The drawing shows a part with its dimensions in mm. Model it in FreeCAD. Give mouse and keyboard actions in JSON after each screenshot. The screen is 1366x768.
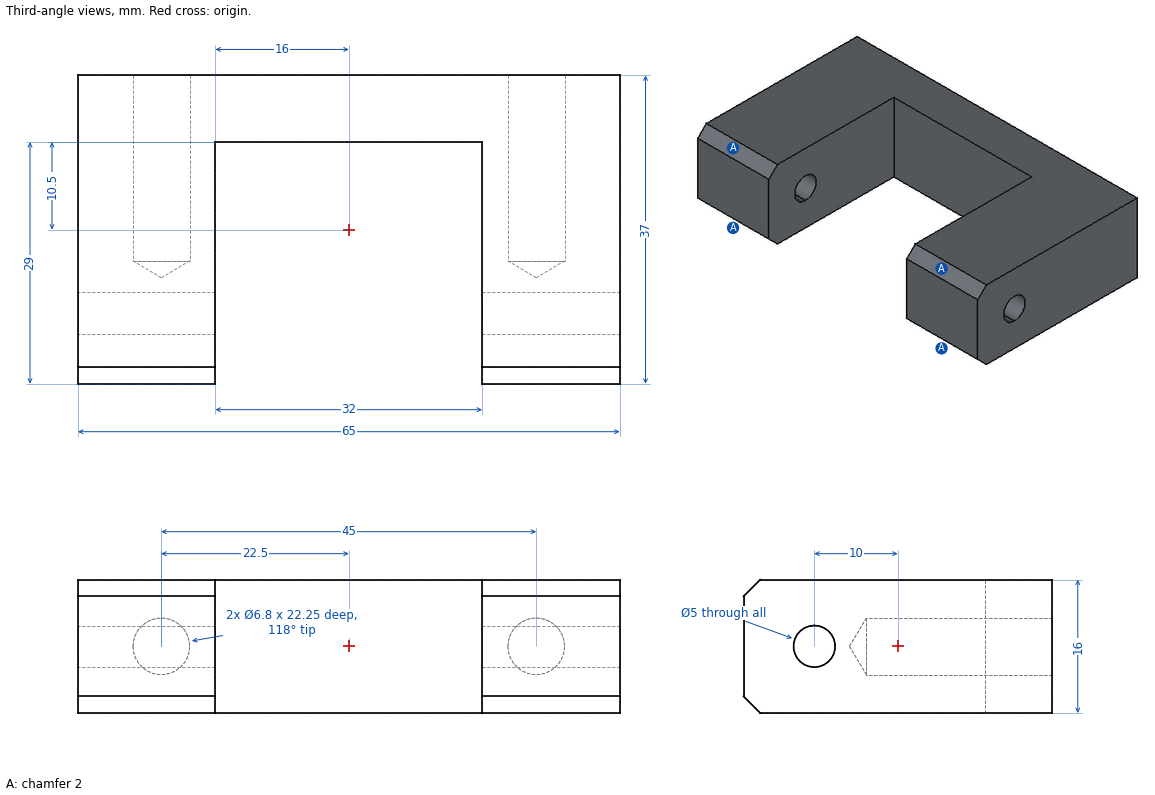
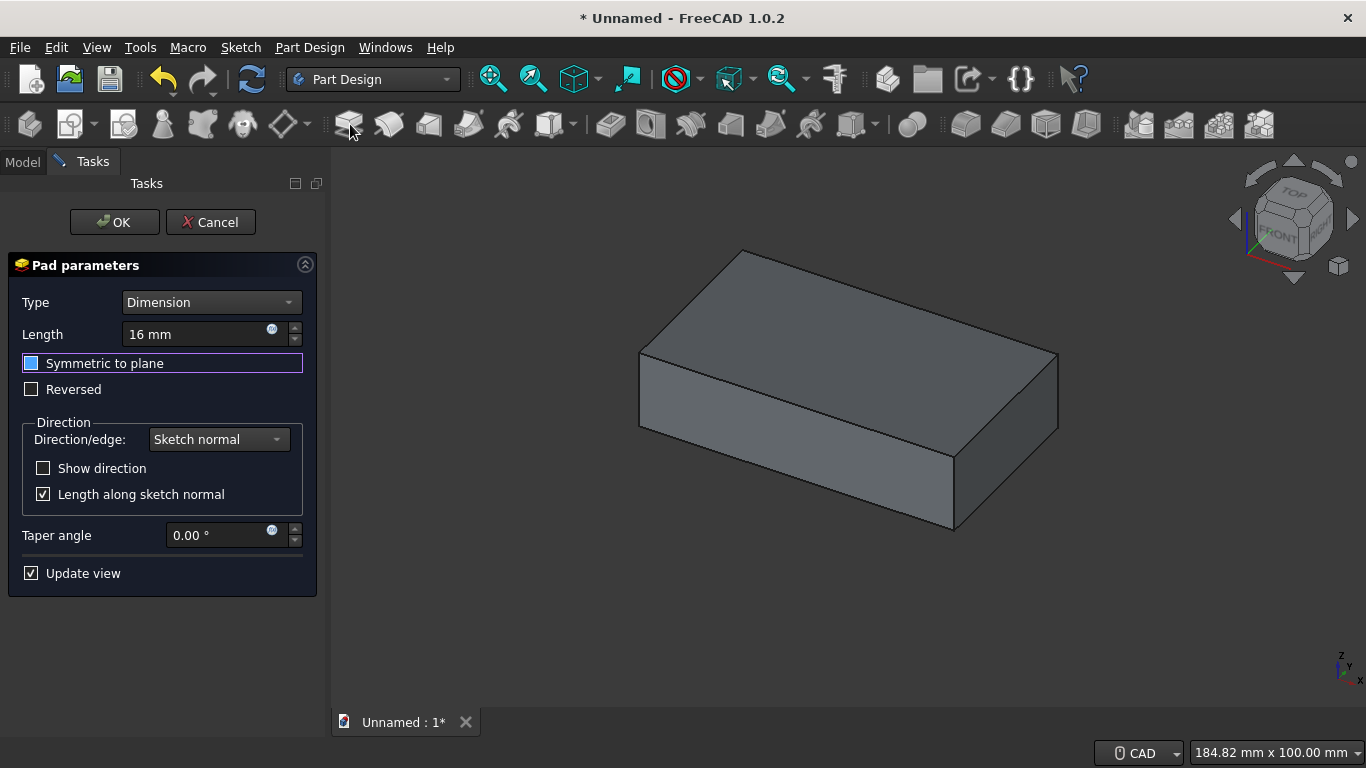
{"action": "left_click", "coordinate": [30, 363]}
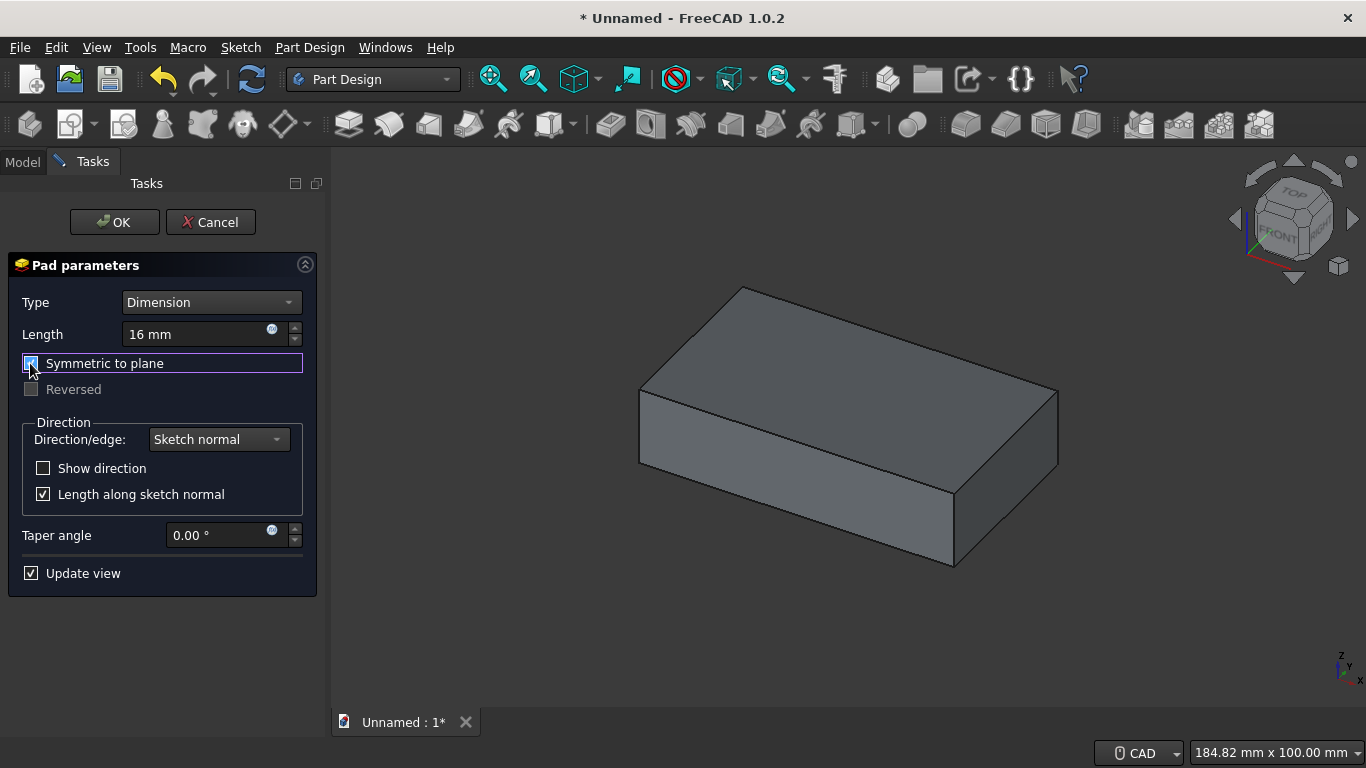
{"action": "left_click", "coordinate": [115, 222]}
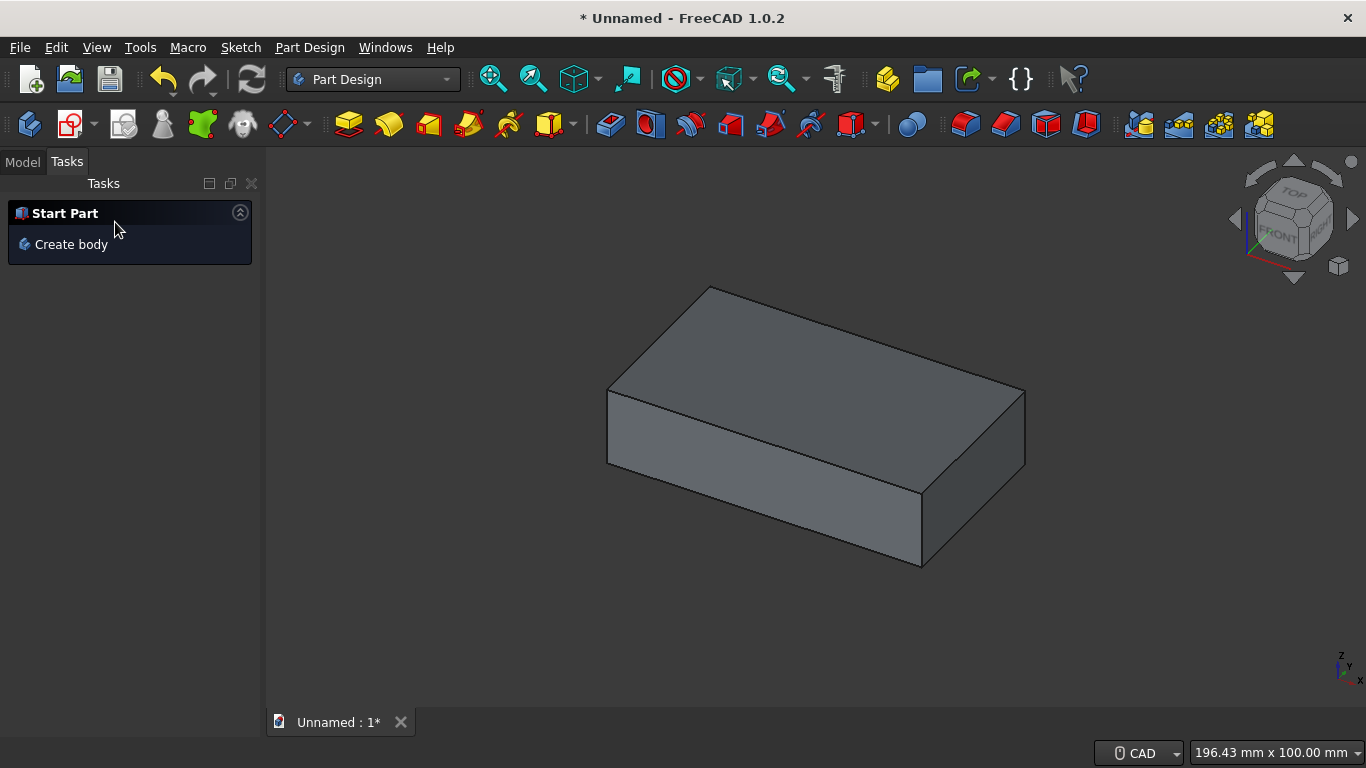
{"action": "left_click", "coordinate": [861, 404]}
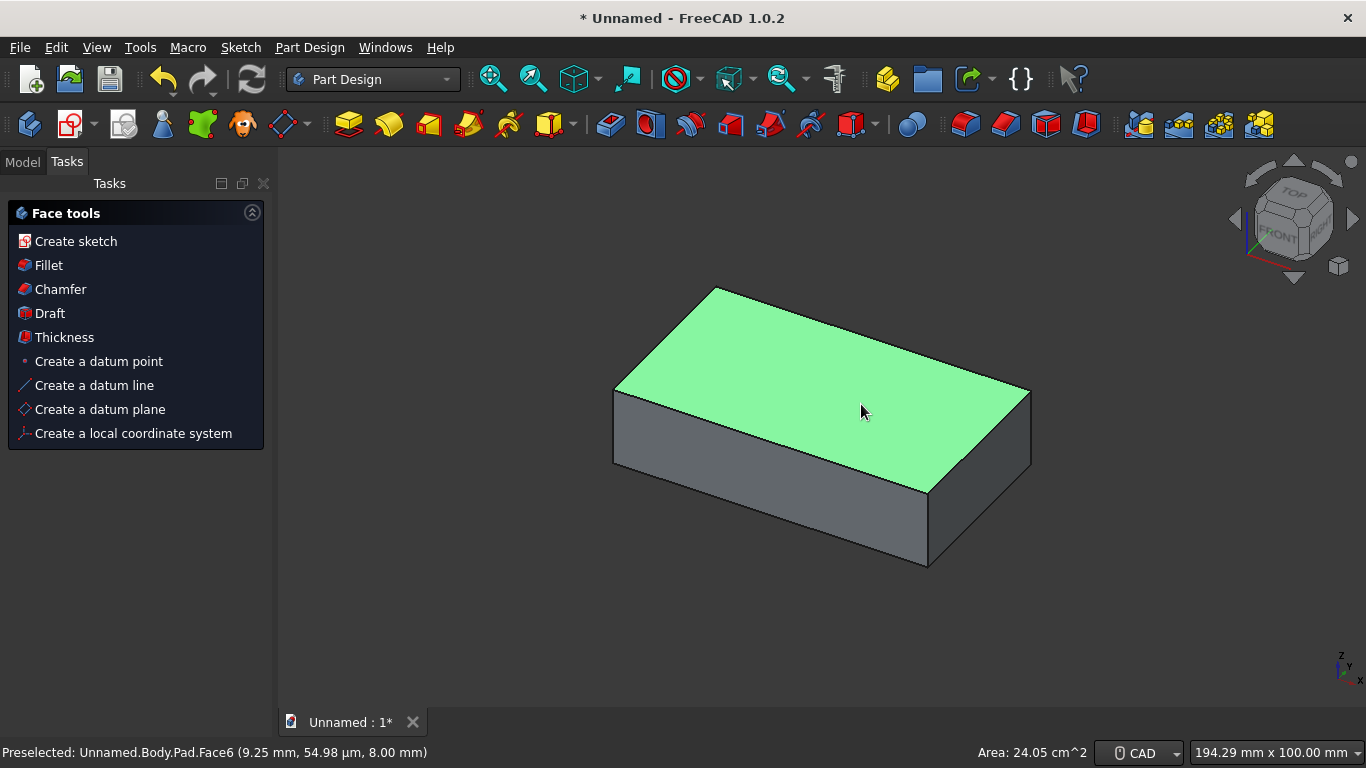
{"action": "left_click", "coordinate": [70, 124]}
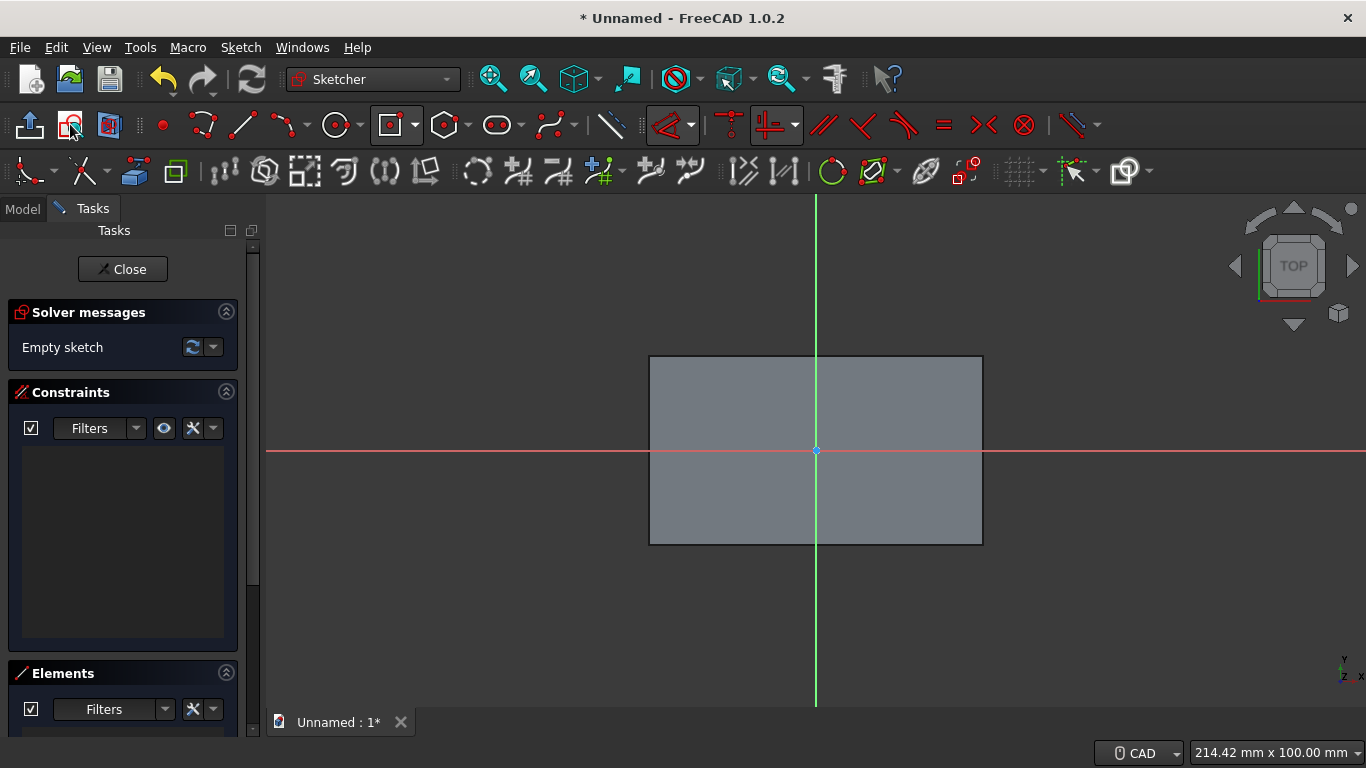
{"action": "scroll", "coordinate": [872, 488], "scroll_direction": "up", "scroll_amount": 4}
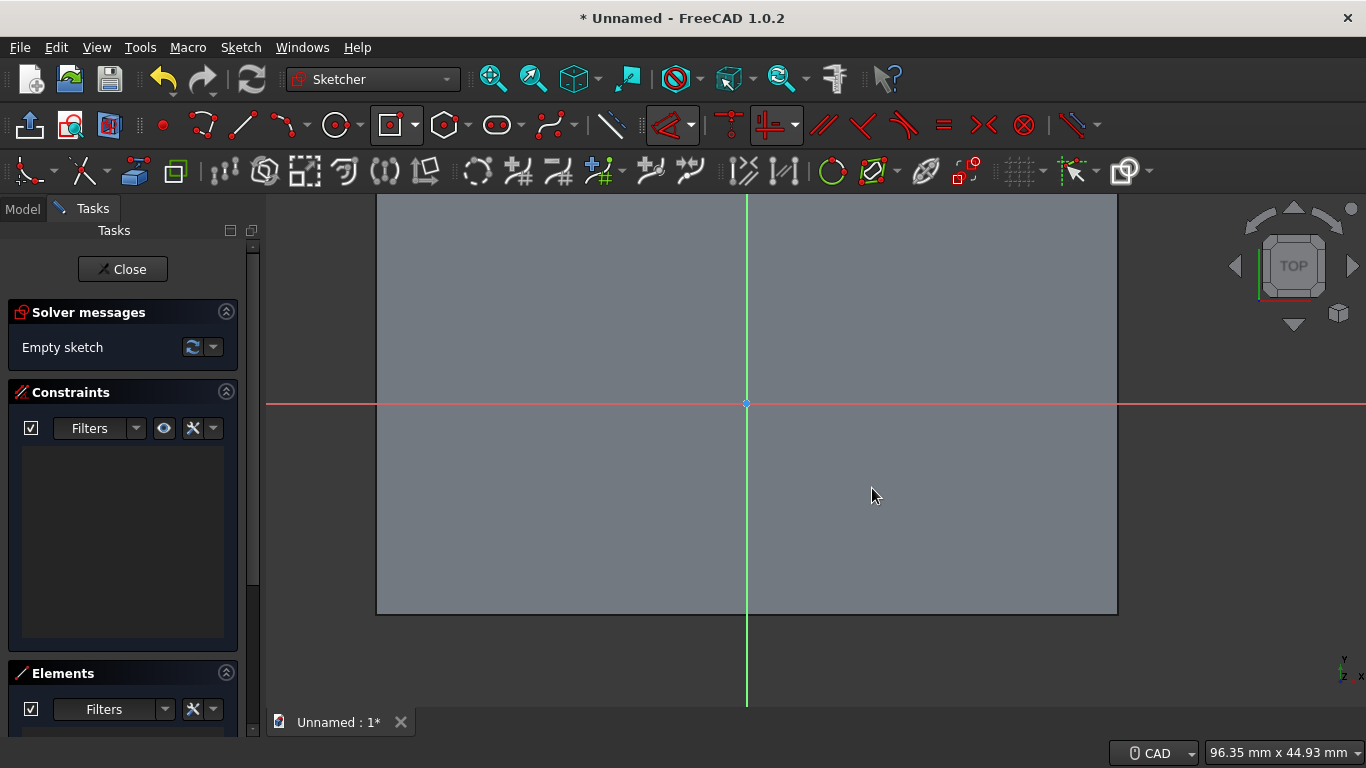
{"action": "key", "text": "g r"}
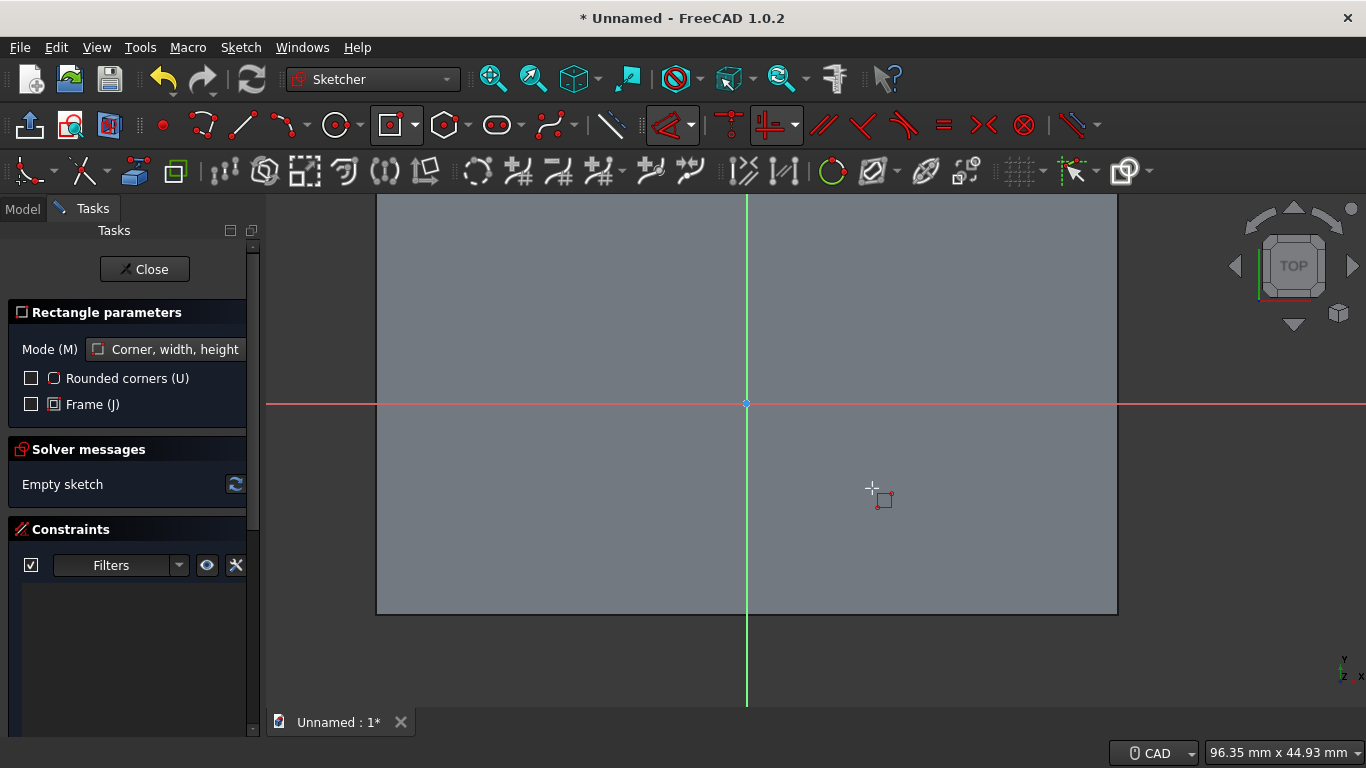
{"action": "left_click", "coordinate": [564, 284]}
{"action": "left_click", "coordinate": [929, 615]}
{"action": "key", "text": "Escape"}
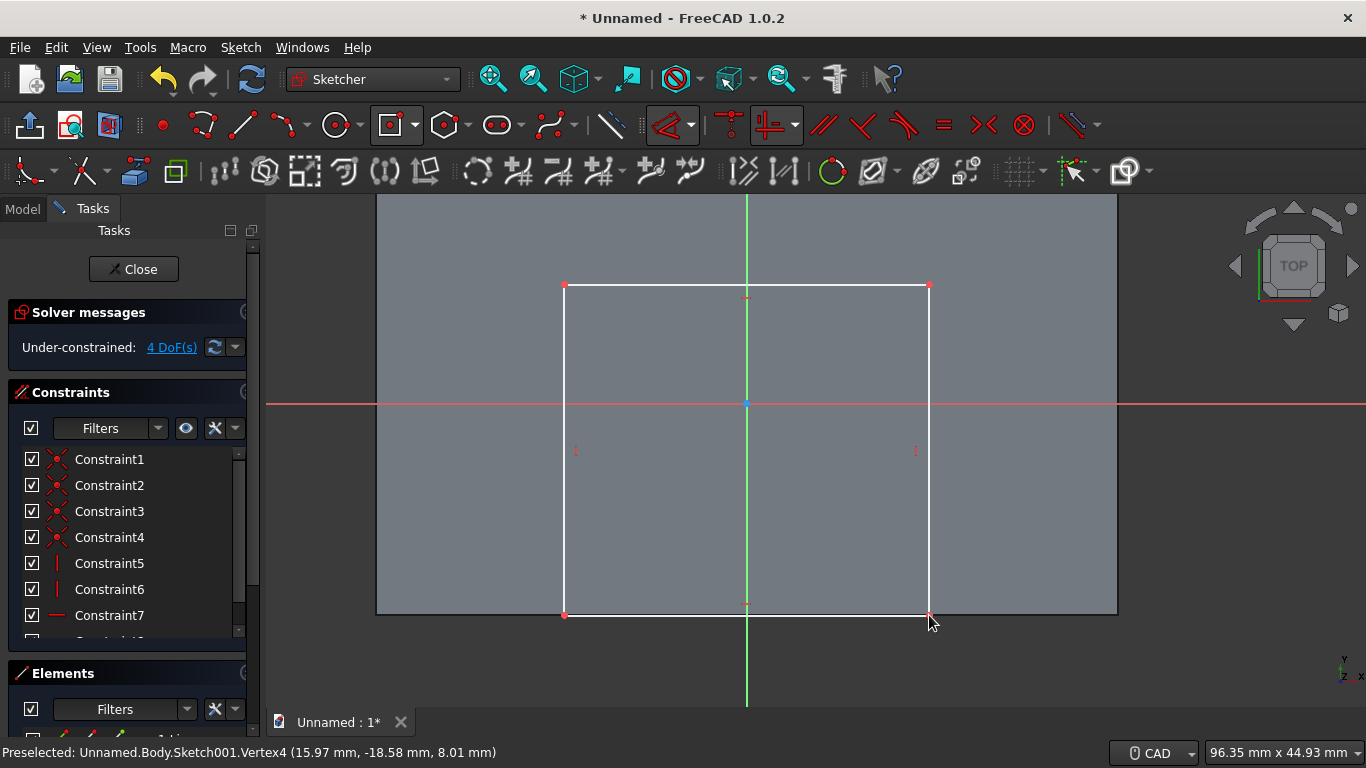
{"action": "left_click", "coordinate": [564, 384]}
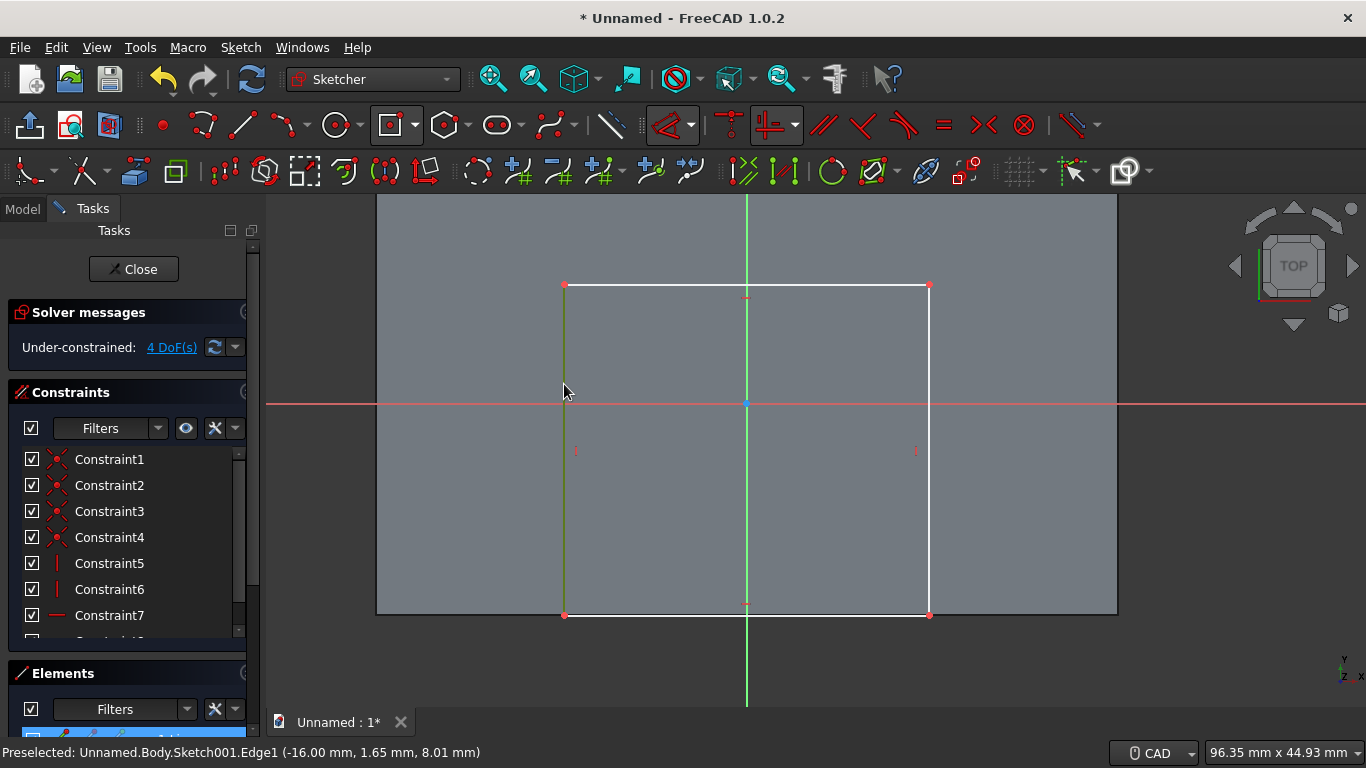
{"action": "left_click", "coordinate": [694, 126]}